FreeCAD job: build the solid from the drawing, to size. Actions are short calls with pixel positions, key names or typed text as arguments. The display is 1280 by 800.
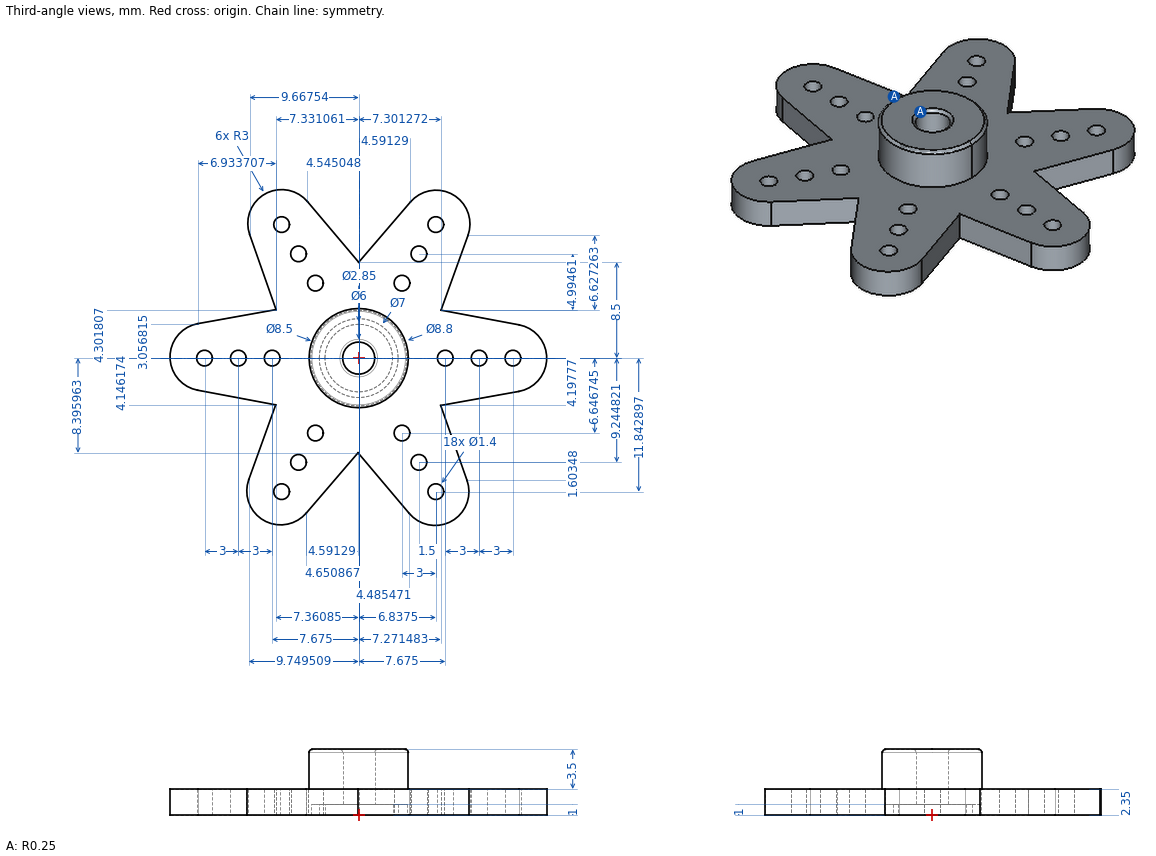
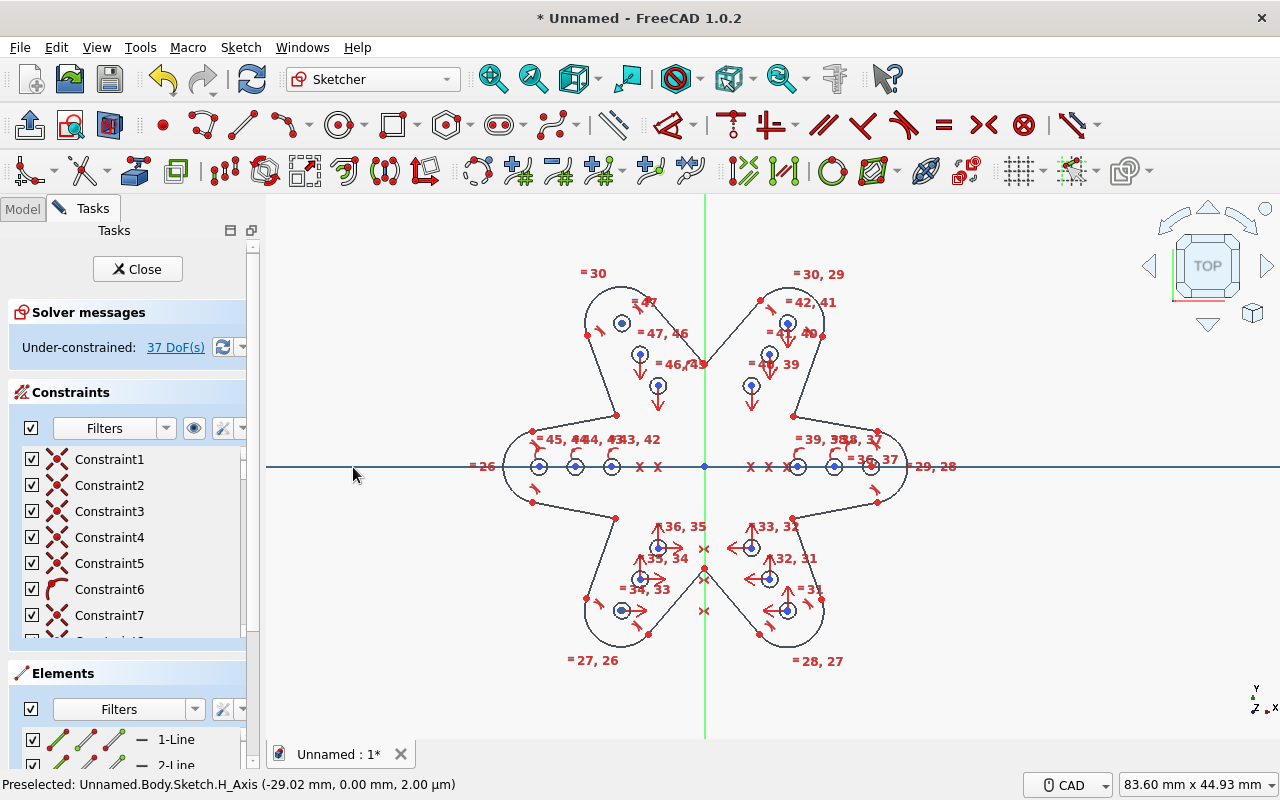
click(984, 126)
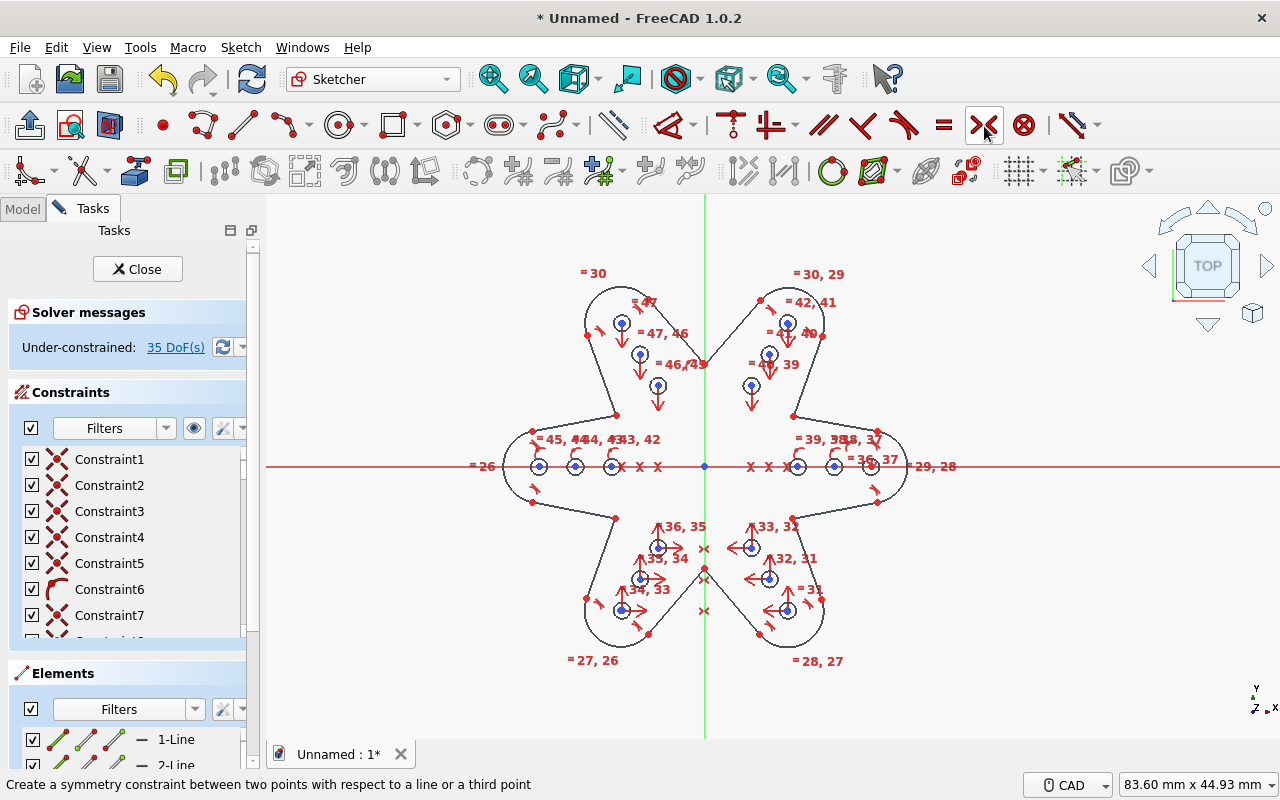
click(668, 126)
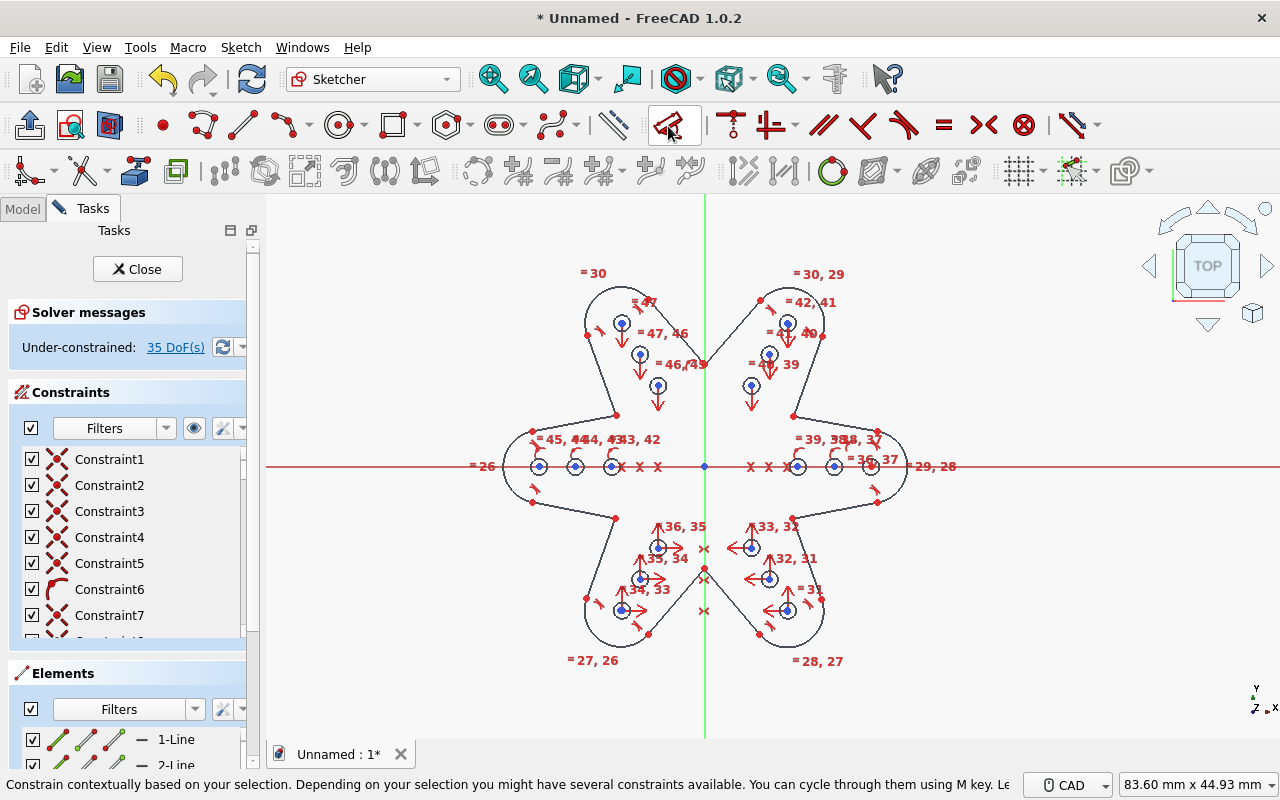
click(509, 448)
click(482, 431)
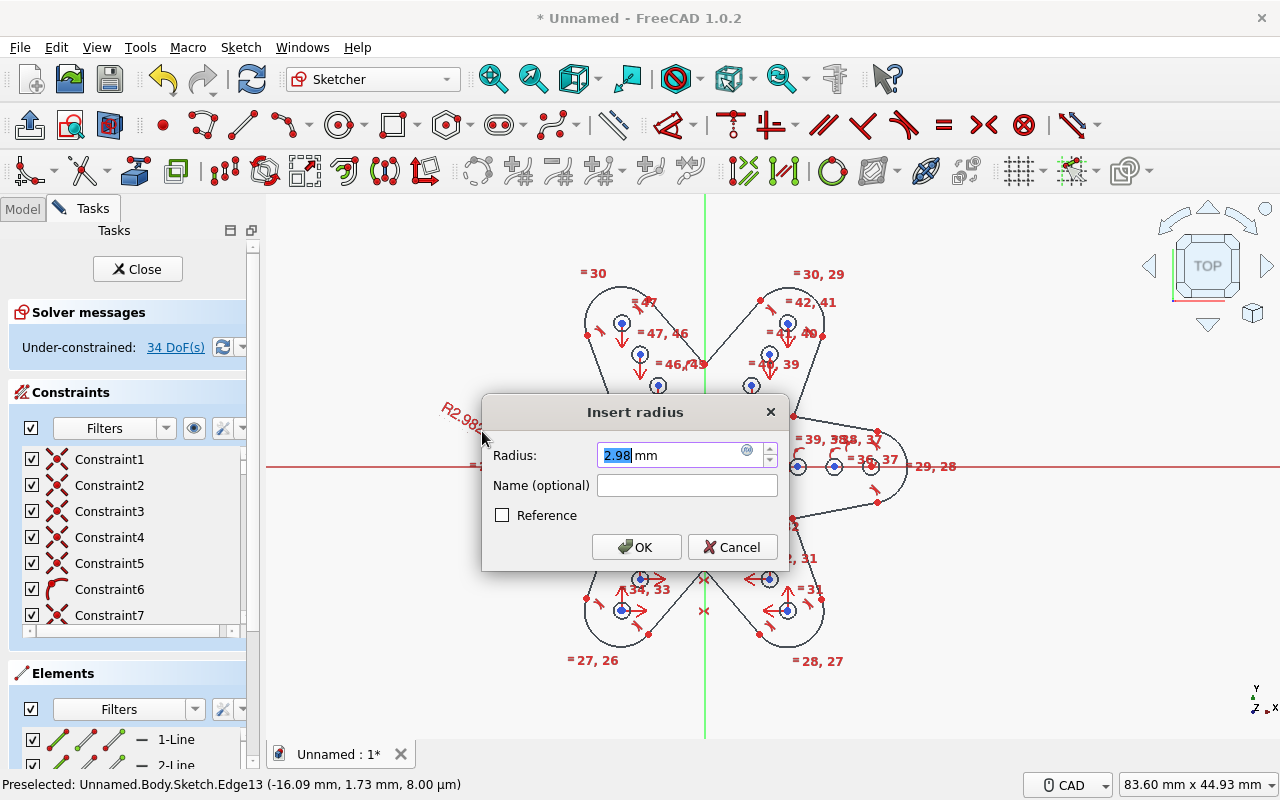
text(3)
key(Return)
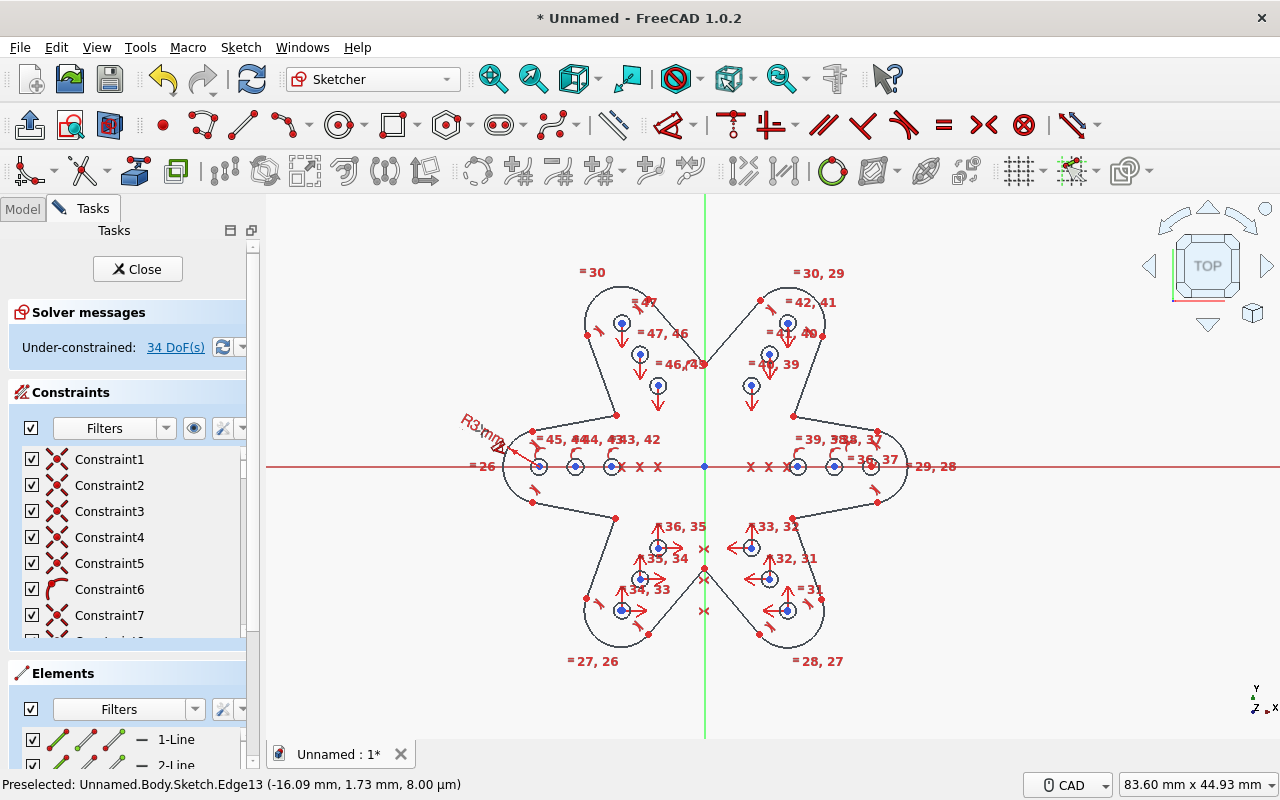
scroll(782, 616, up, 5)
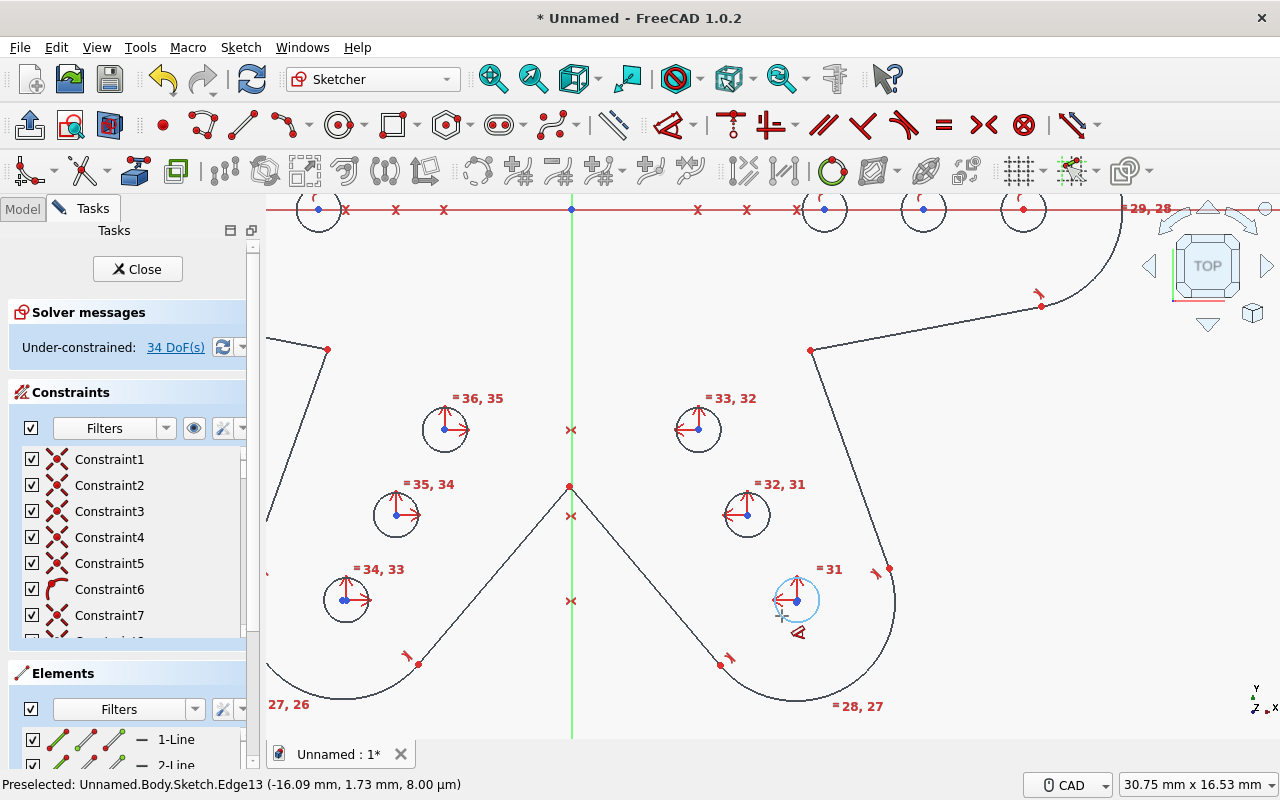
click(782, 616)
click(760, 639)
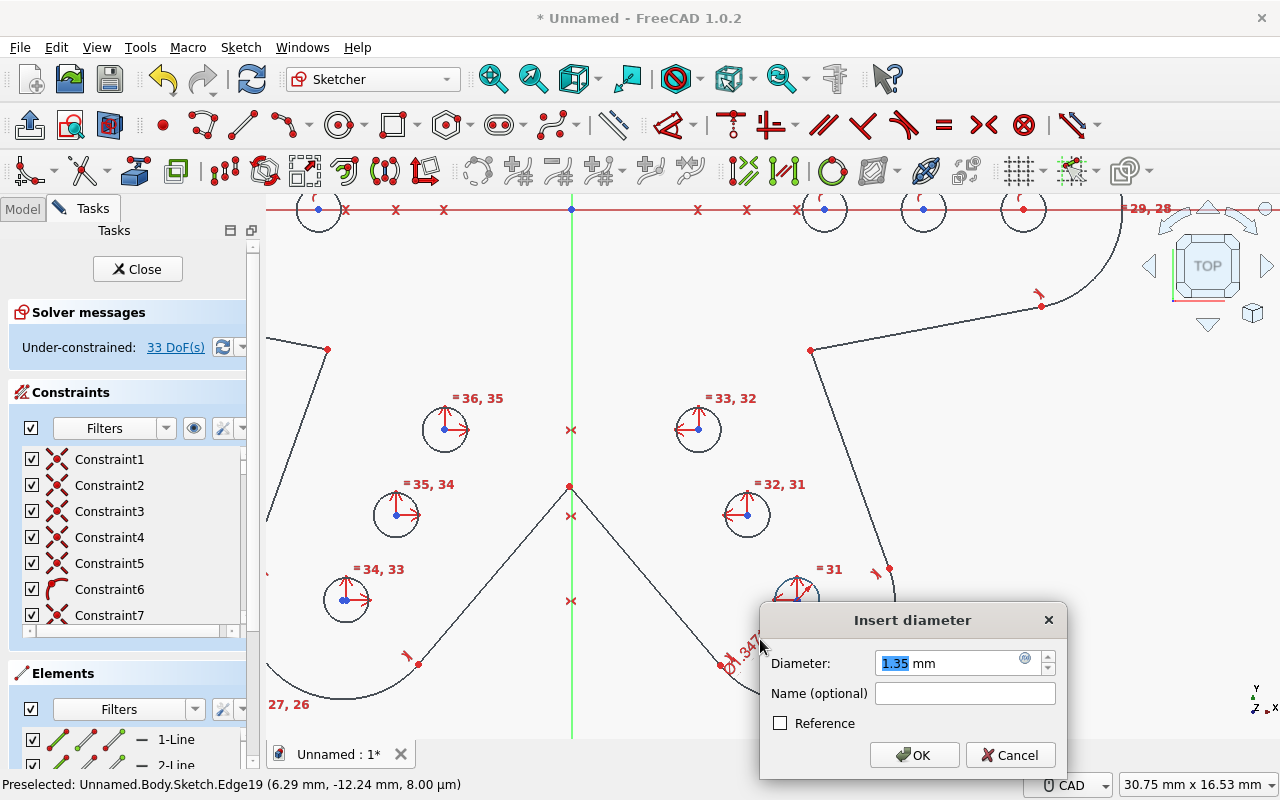
text(1.4)
key(Return)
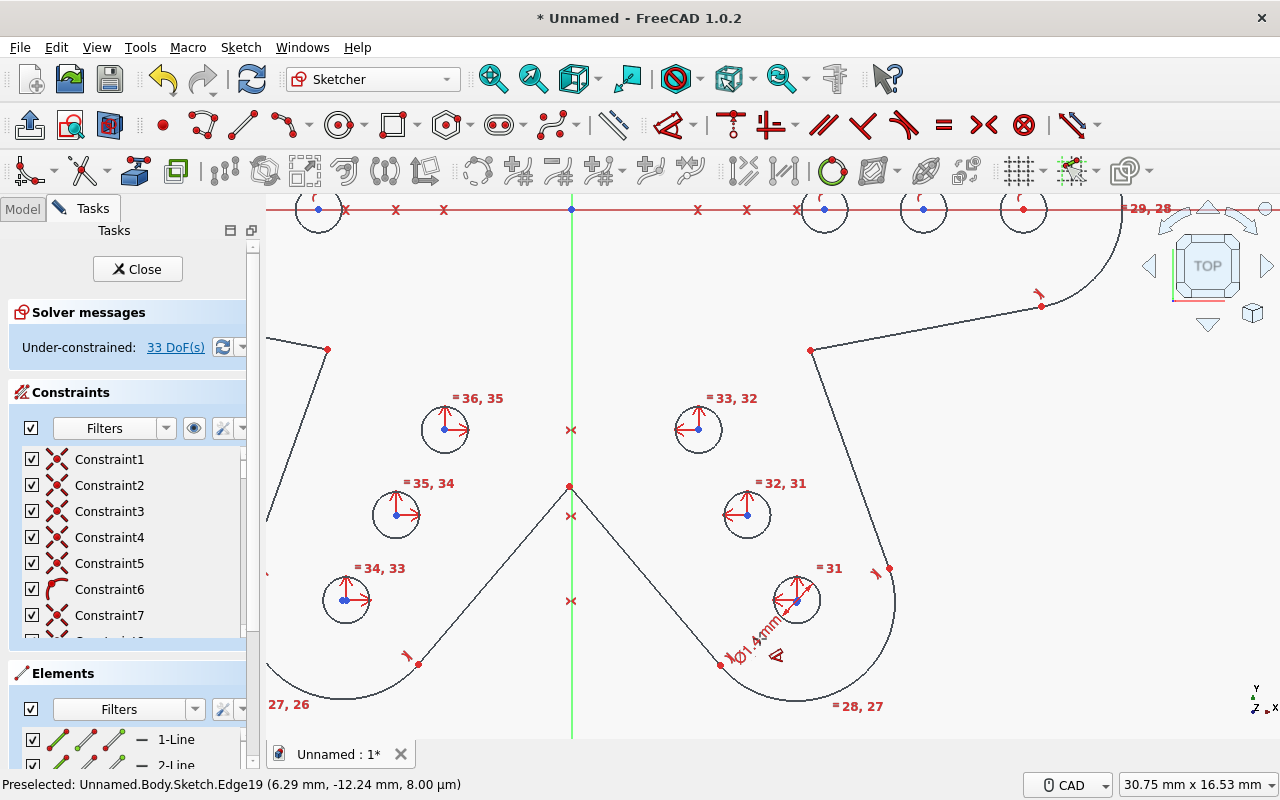
scroll(797, 600, up, 9)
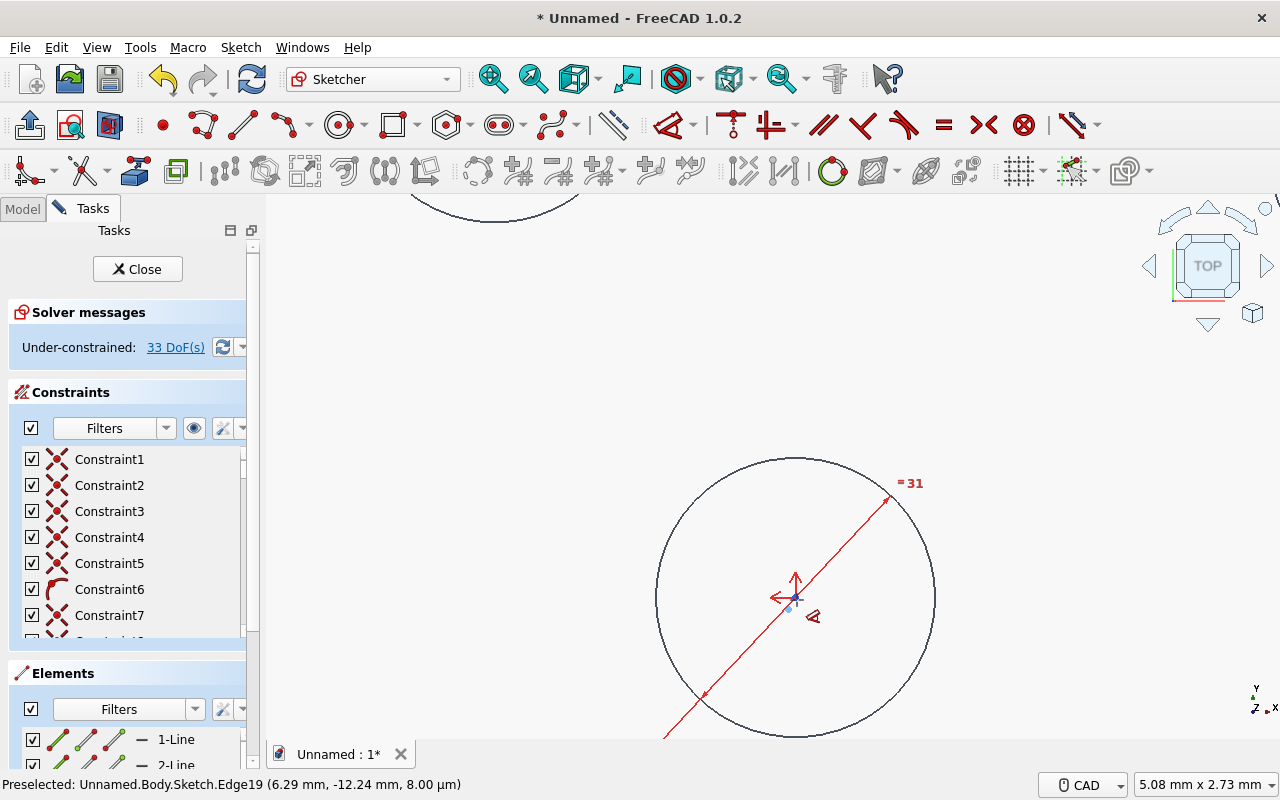
click(796, 598)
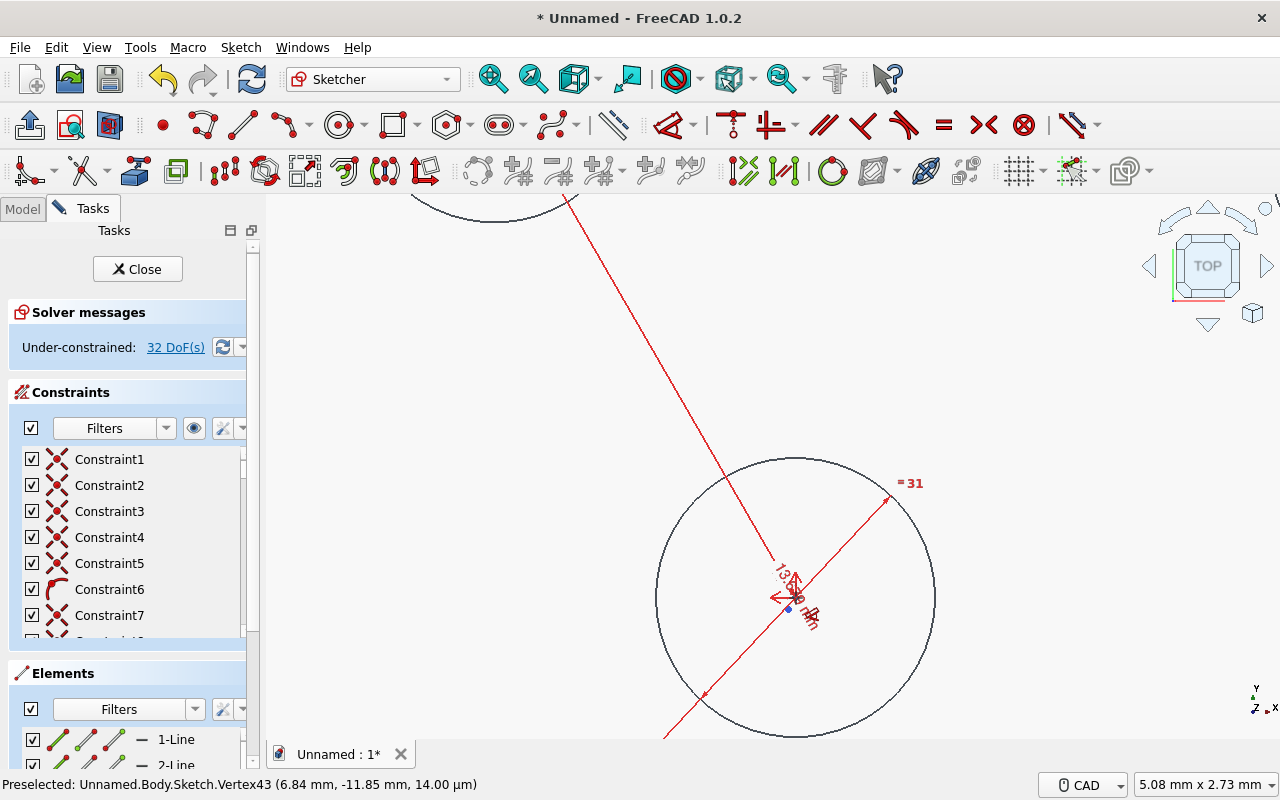
scroll(787, 612, down, 14)